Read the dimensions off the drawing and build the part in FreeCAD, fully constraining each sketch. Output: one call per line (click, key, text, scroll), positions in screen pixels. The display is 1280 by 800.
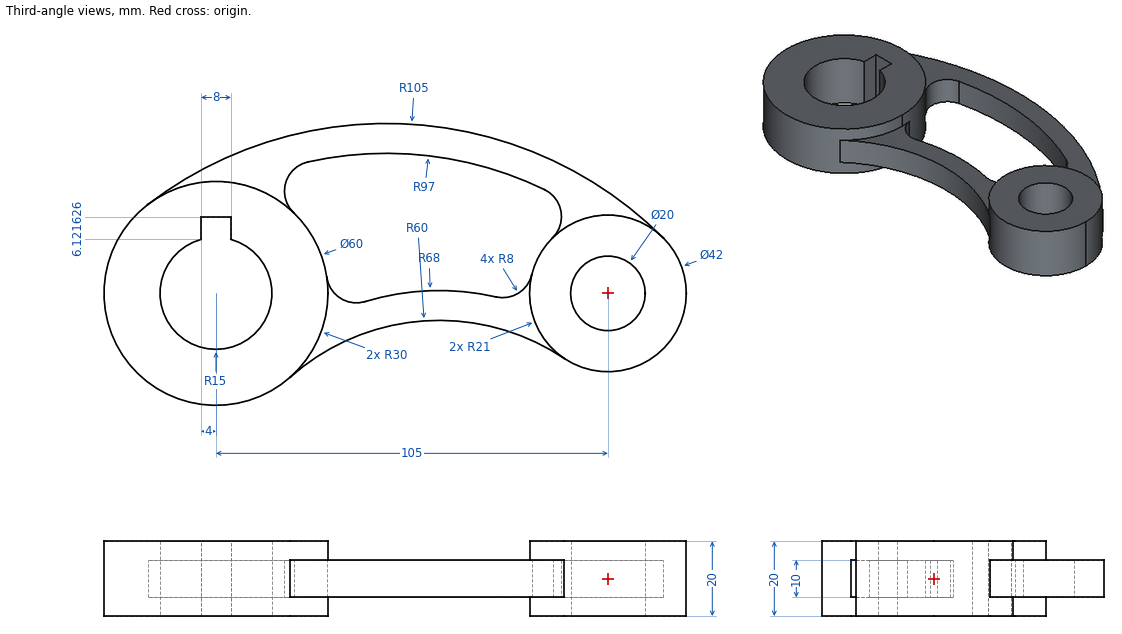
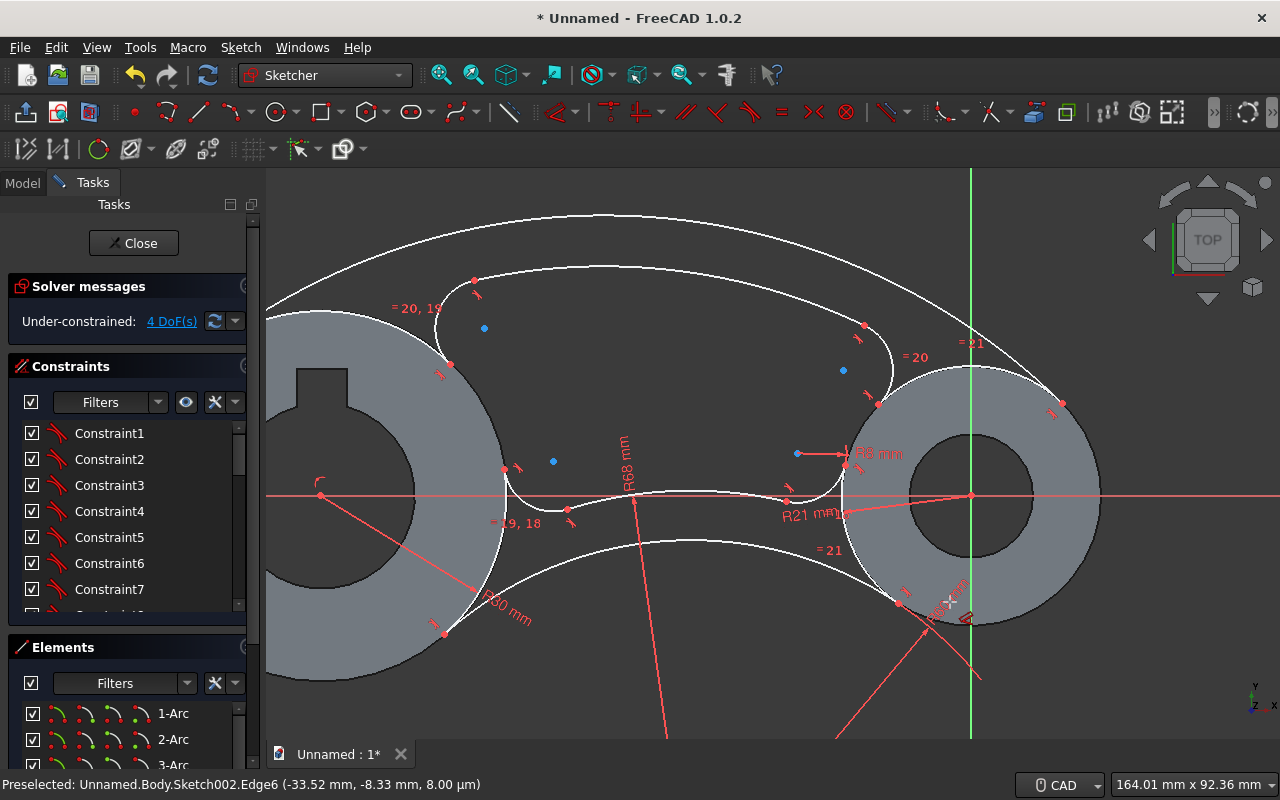
click(828, 255)
click(839, 225)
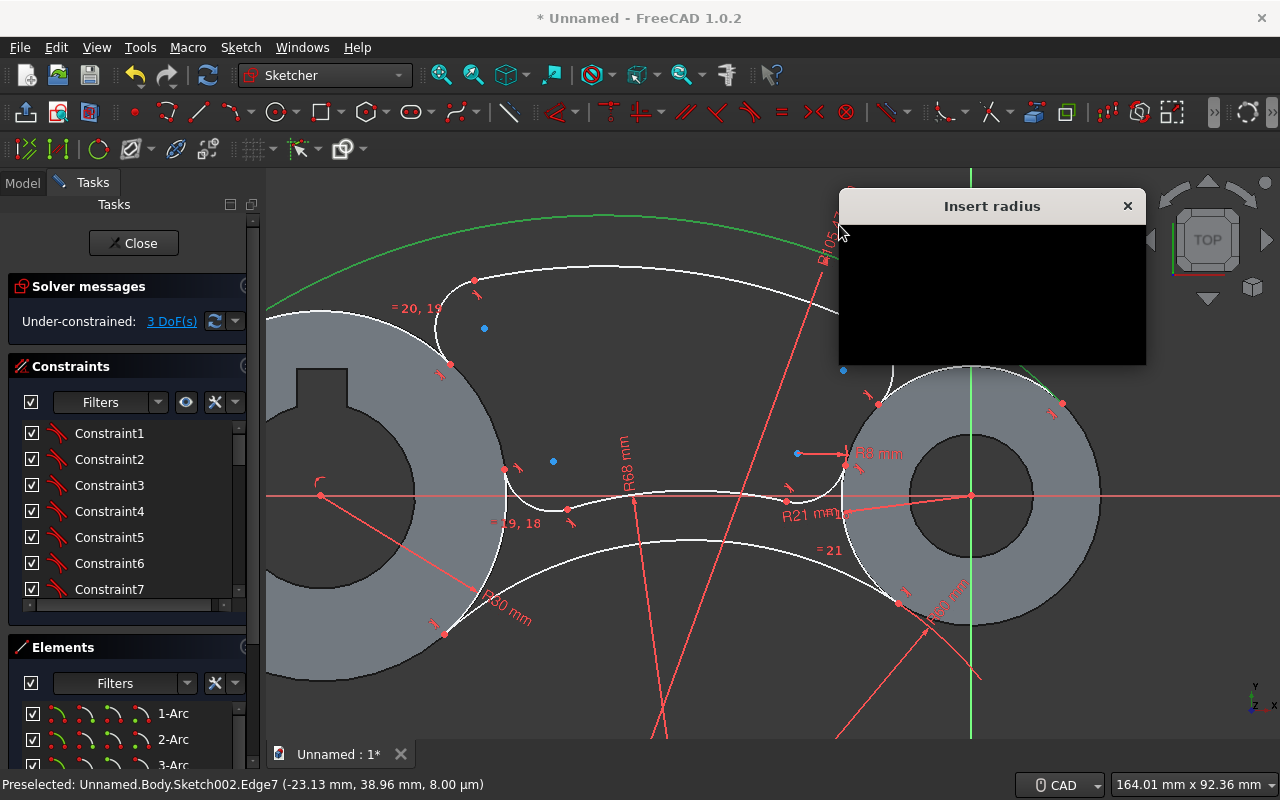
text(105)
key(Return)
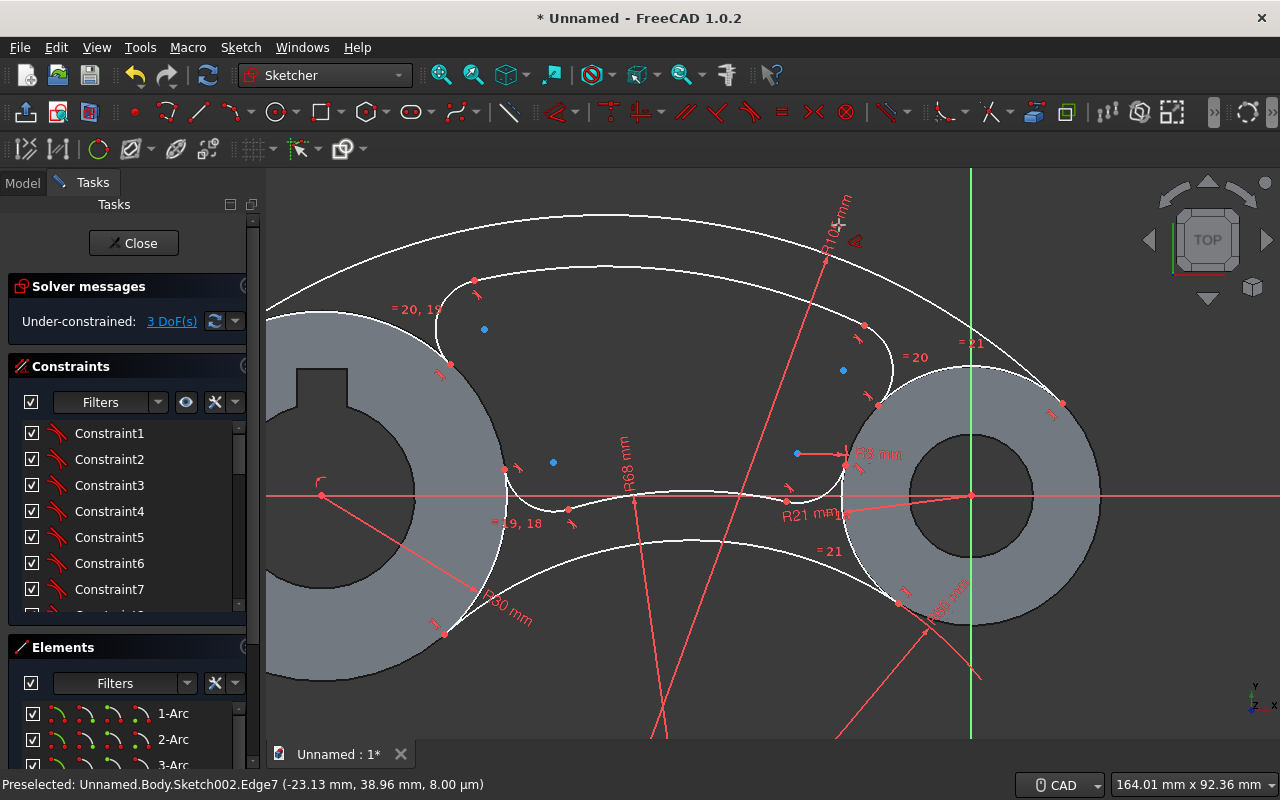
click(384, 323)
click(395, 293)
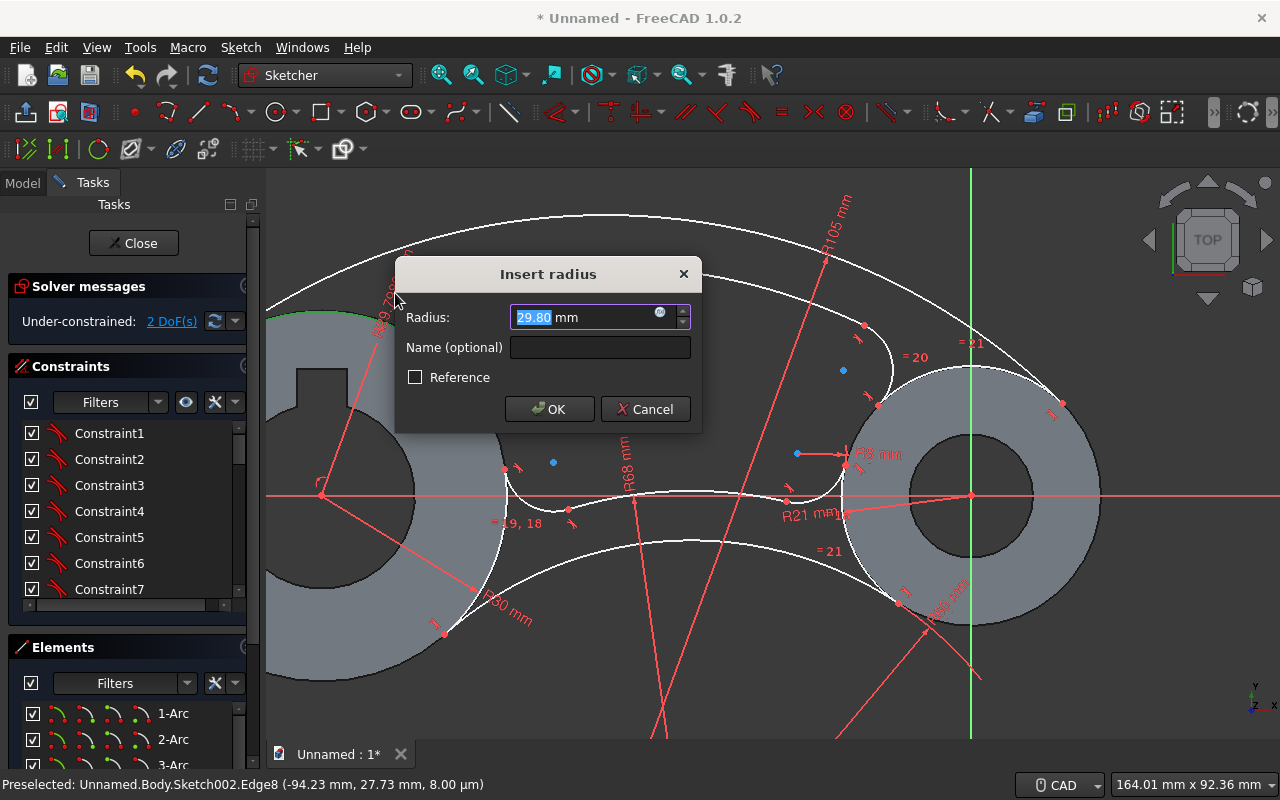
text(30)
key(Return)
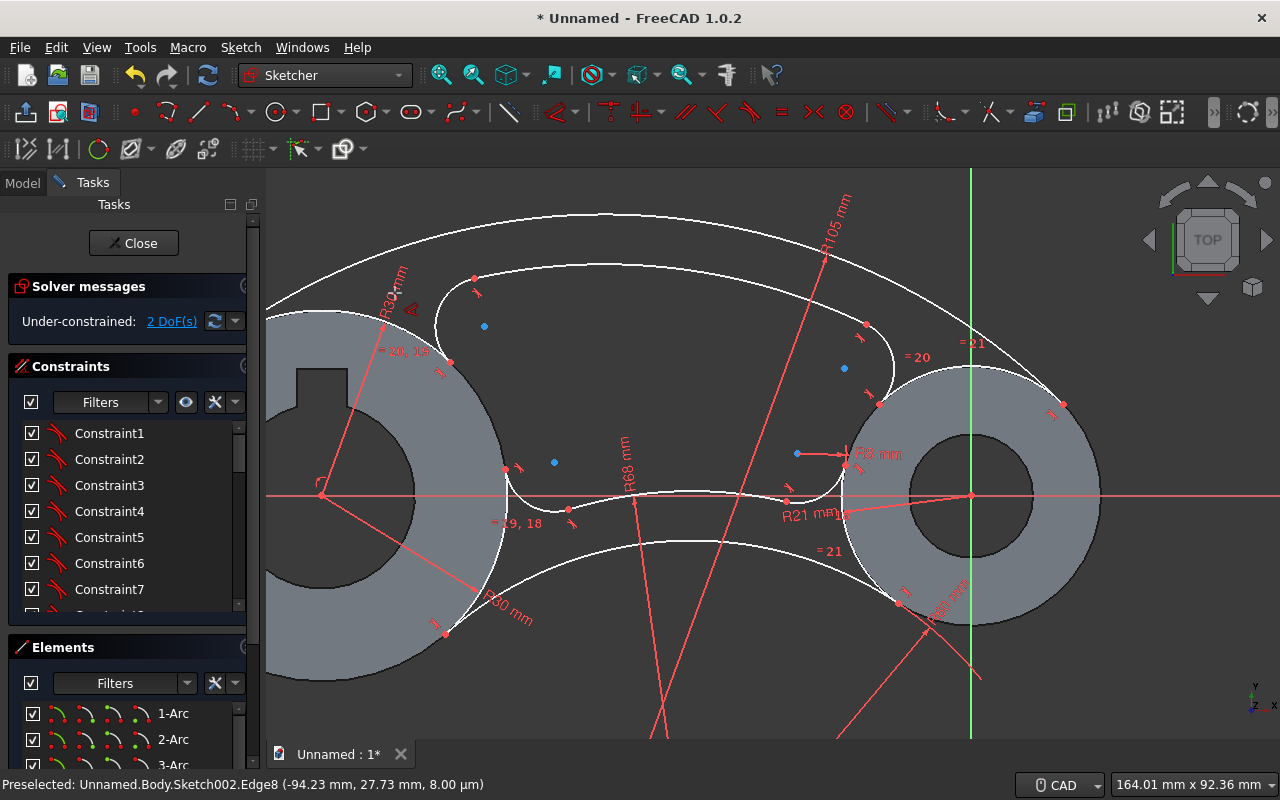
click(753, 283)
click(761, 252)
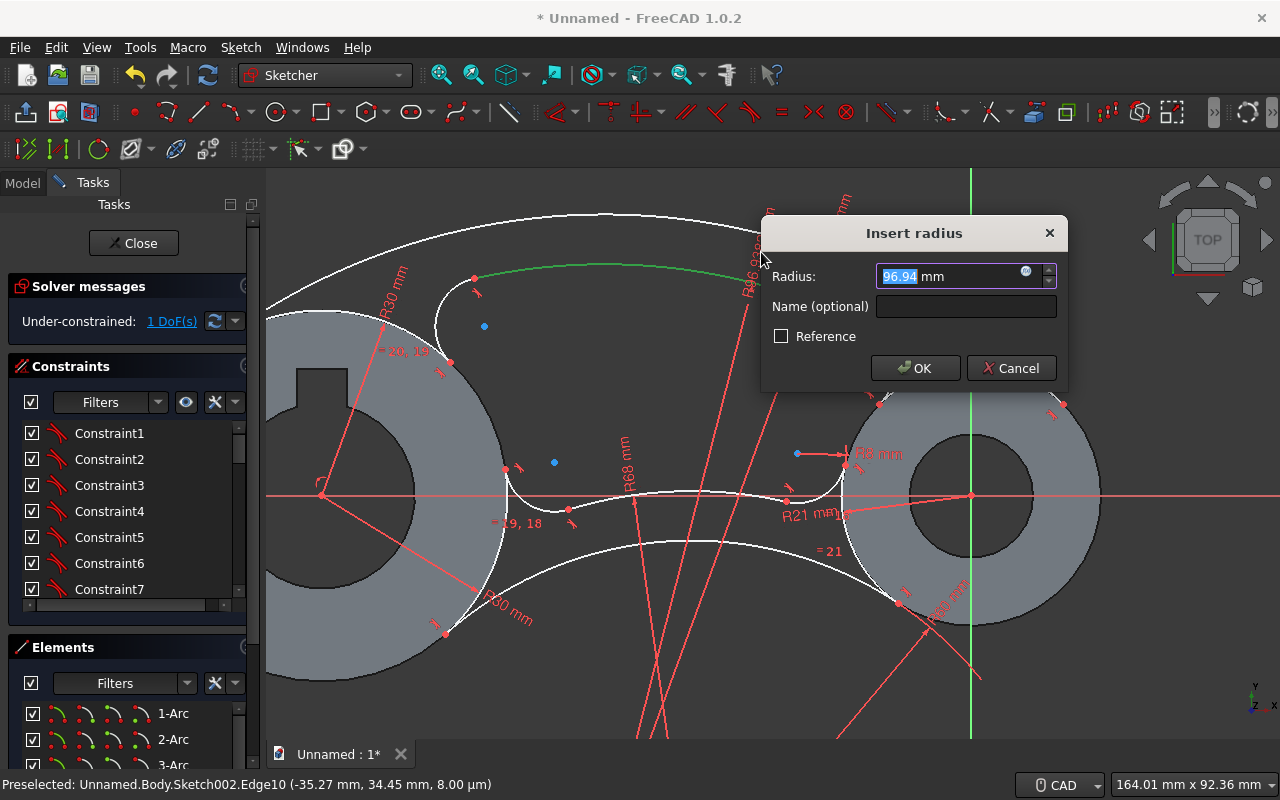
text(97)
key(Return)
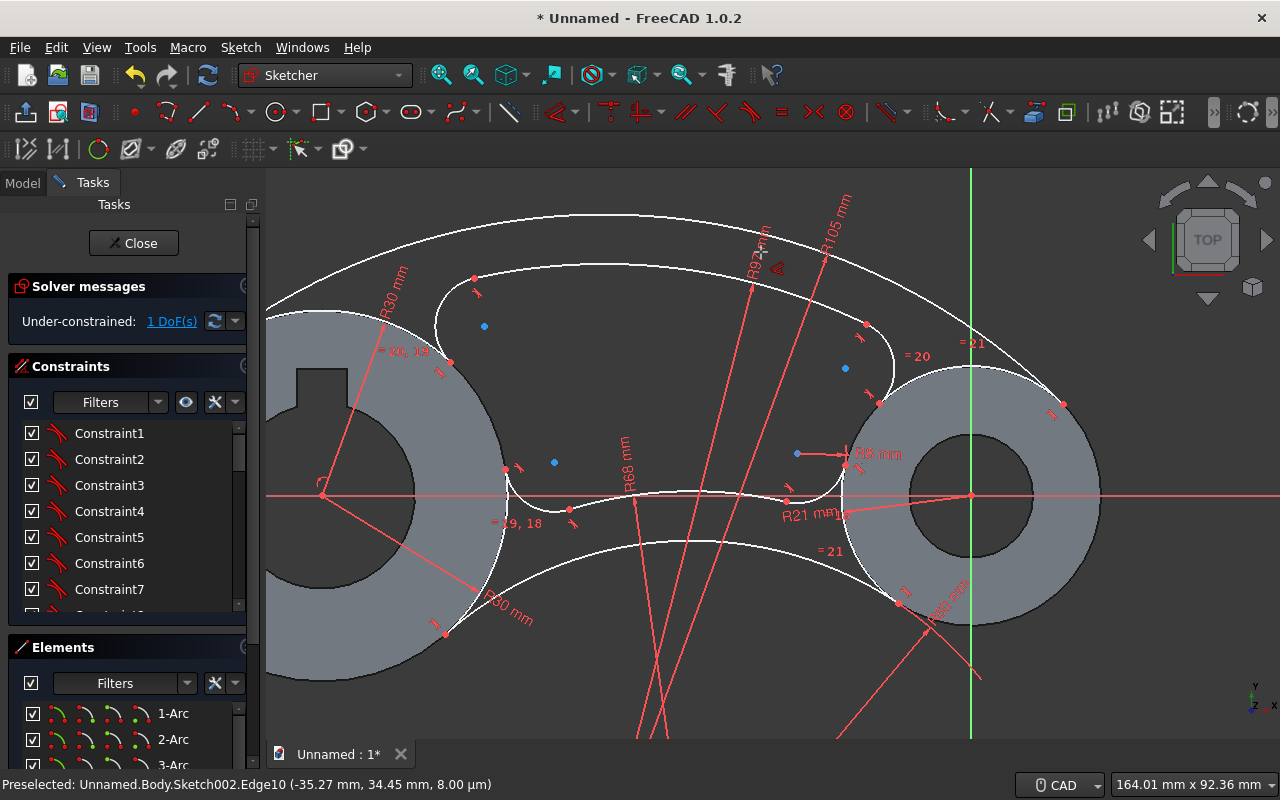
click(322, 496)
click(647, 530)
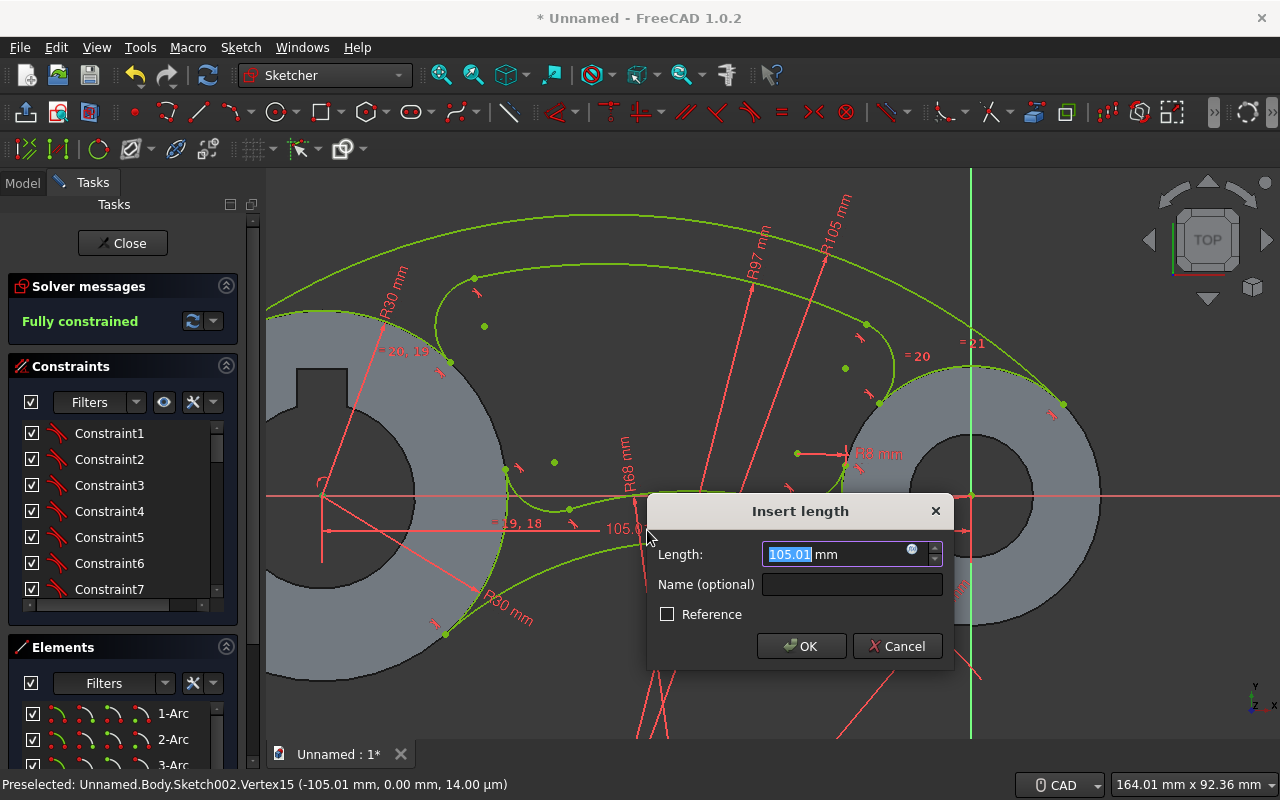
text(105)
key(Return)
key(Escape)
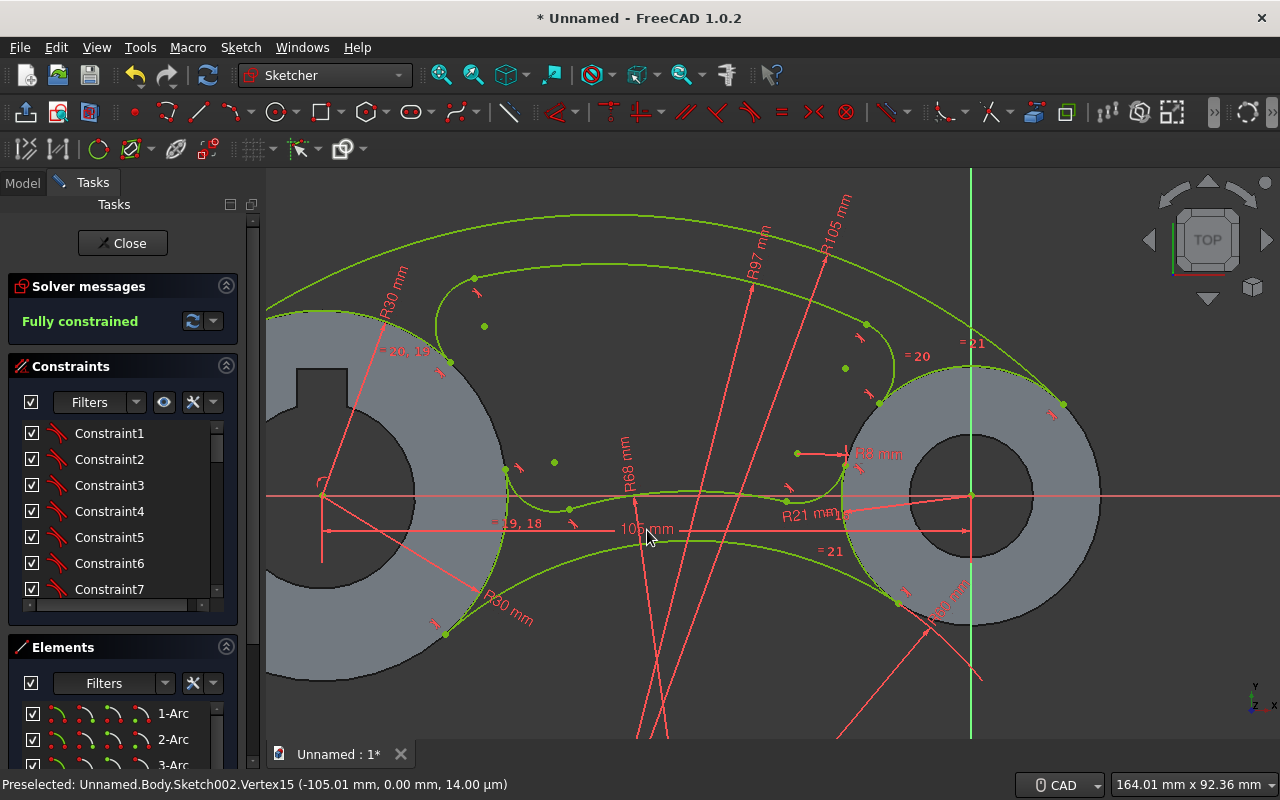
click(123, 243)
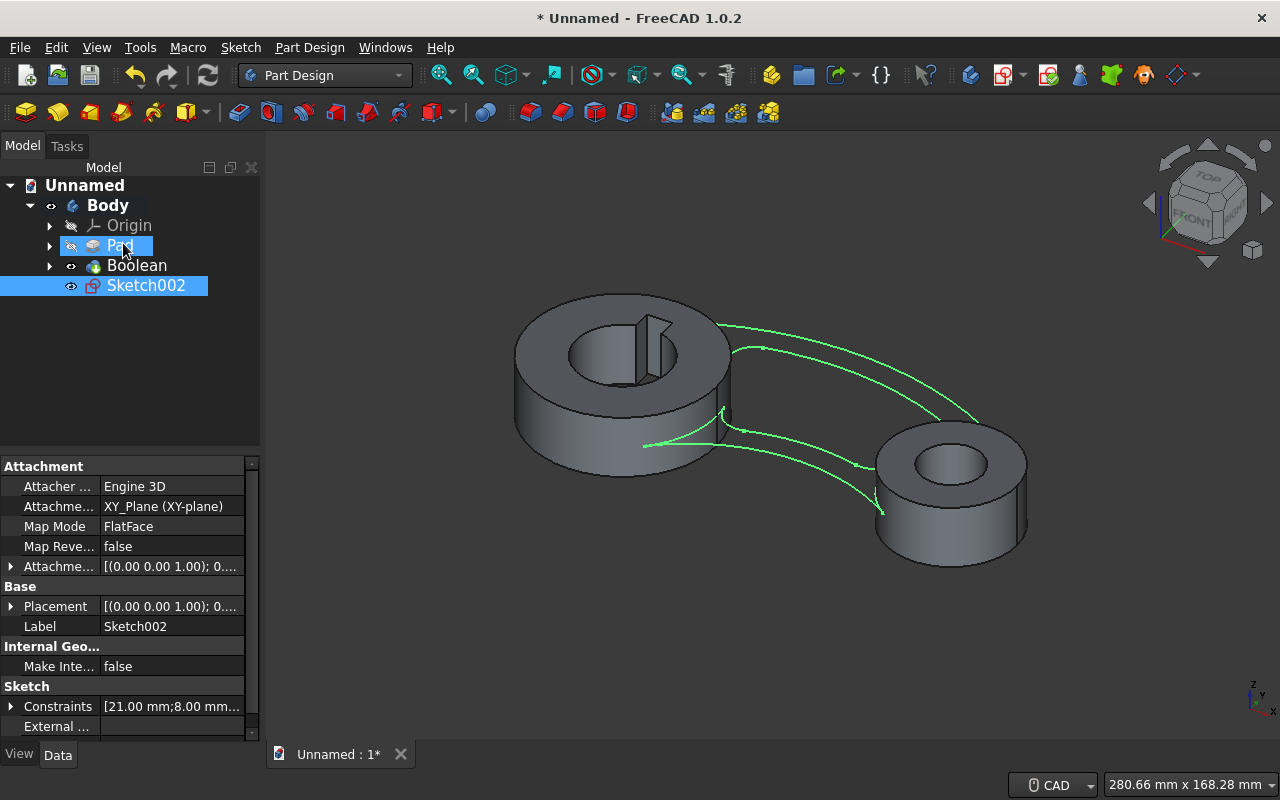
click(26, 112)